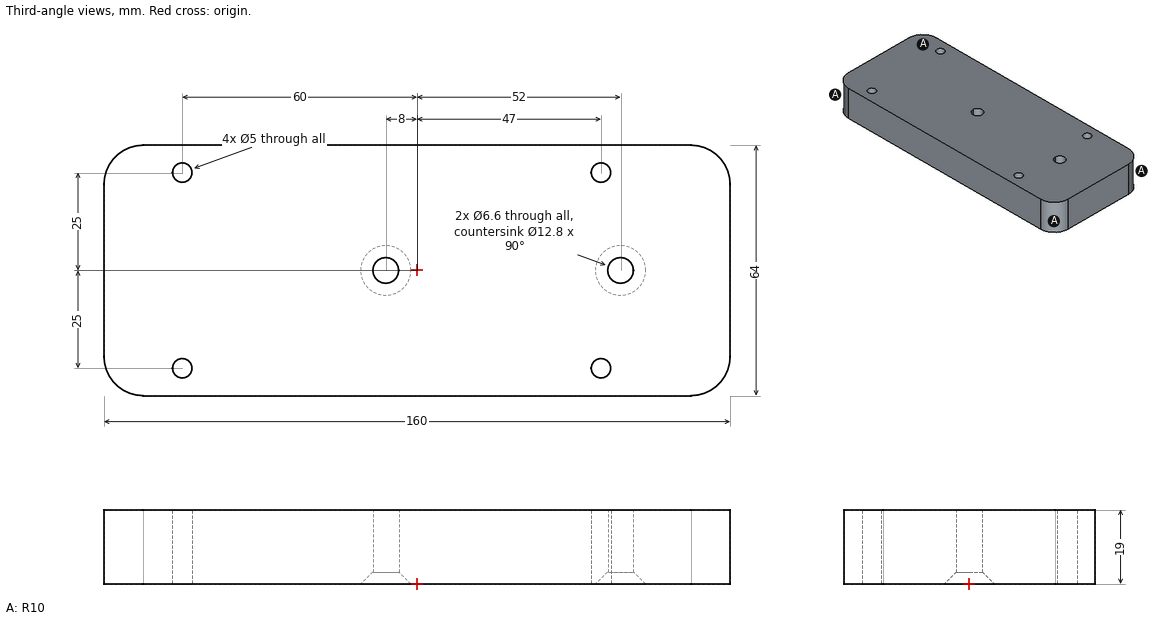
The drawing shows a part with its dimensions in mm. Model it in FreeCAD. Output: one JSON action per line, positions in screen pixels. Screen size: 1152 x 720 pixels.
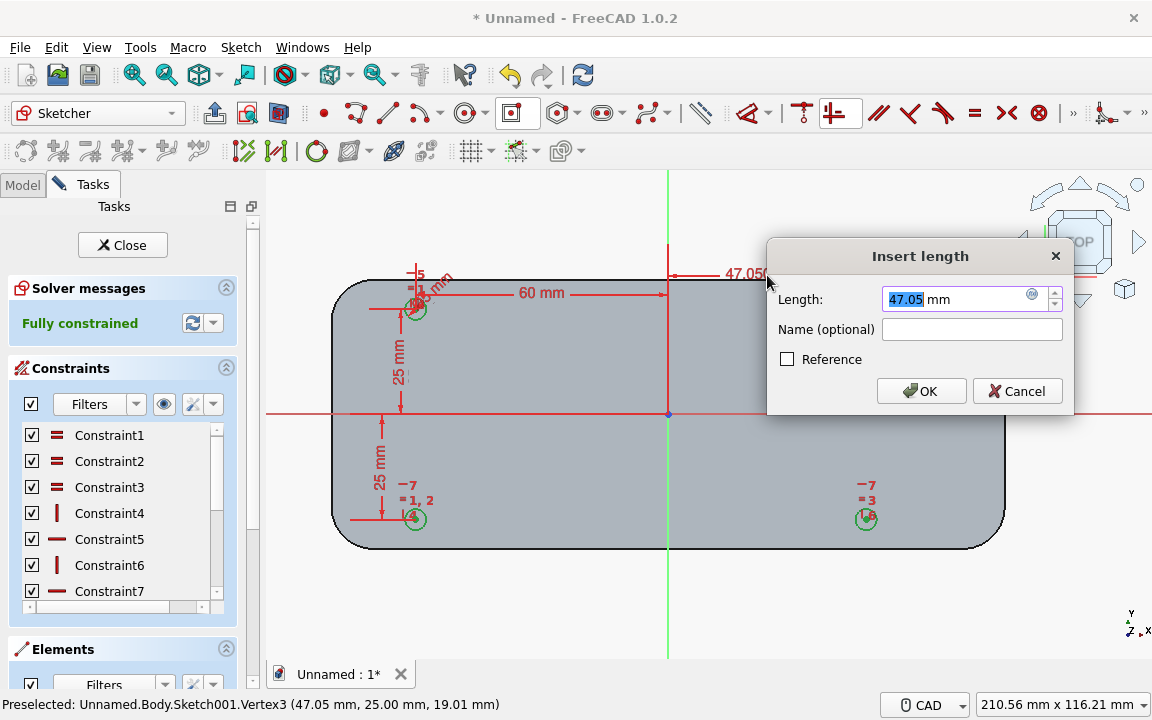
{"action": "type", "text": "47"}
{"action": "key", "text": "Return"}
{"action": "key", "text": "Escape"}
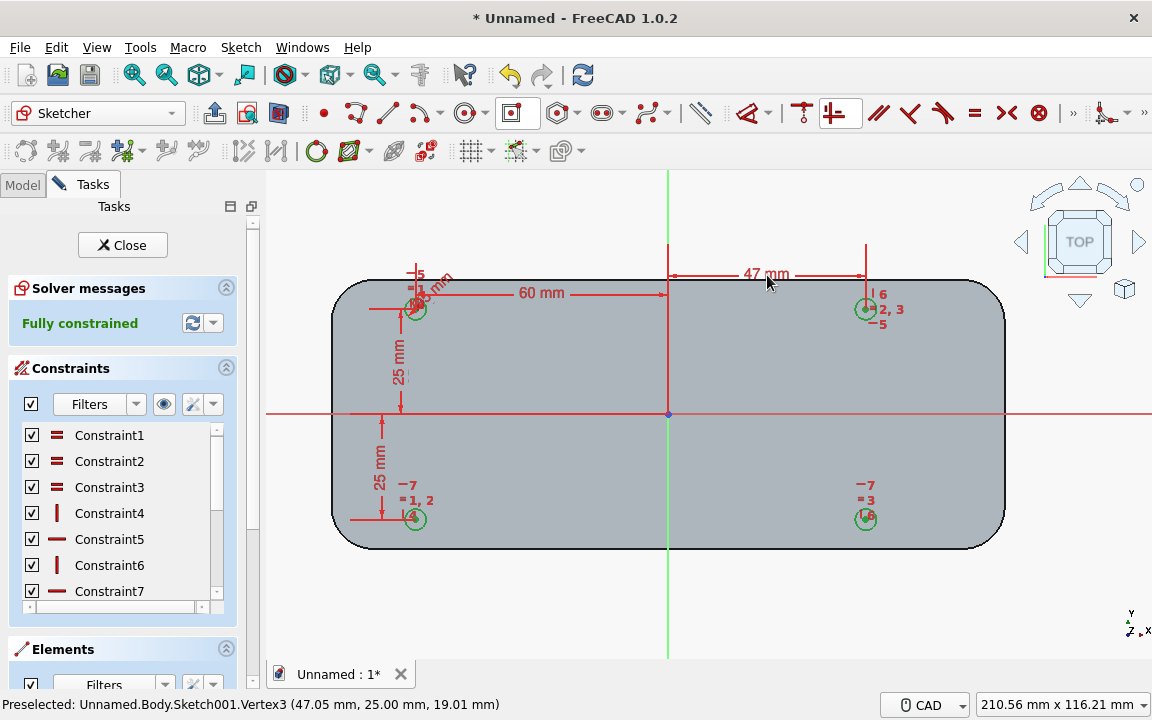
{"action": "left_click", "coordinate": [123, 245]}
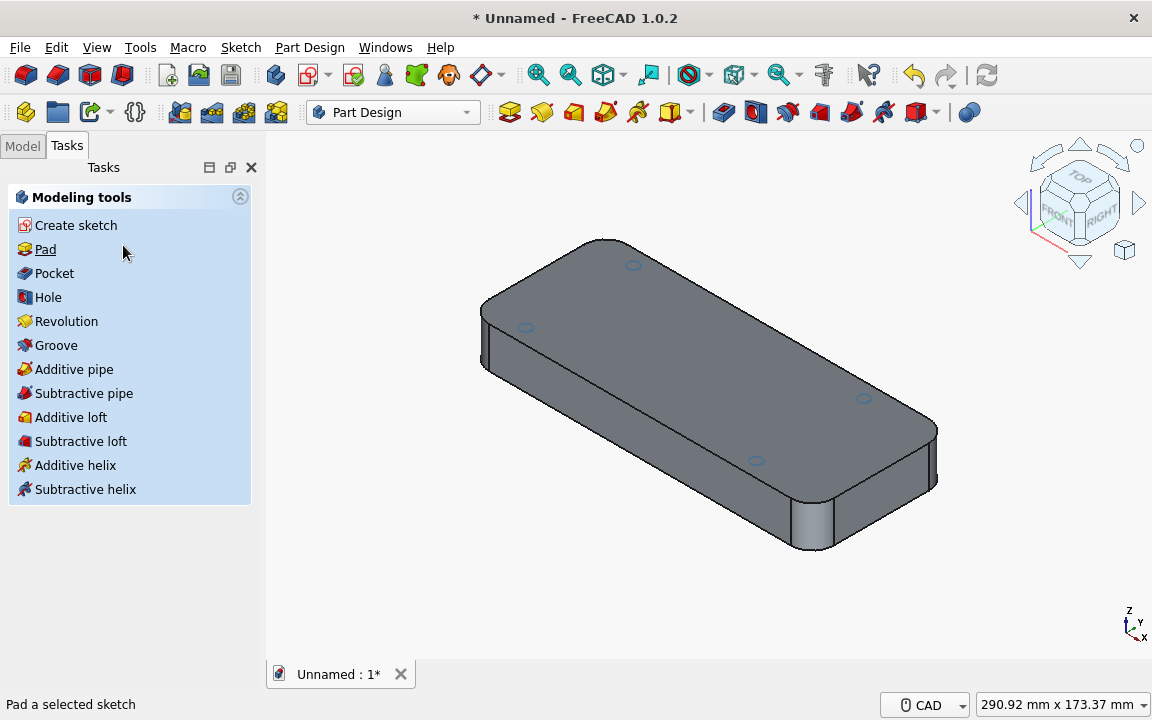
{"action": "left_click", "coordinate": [756, 112]}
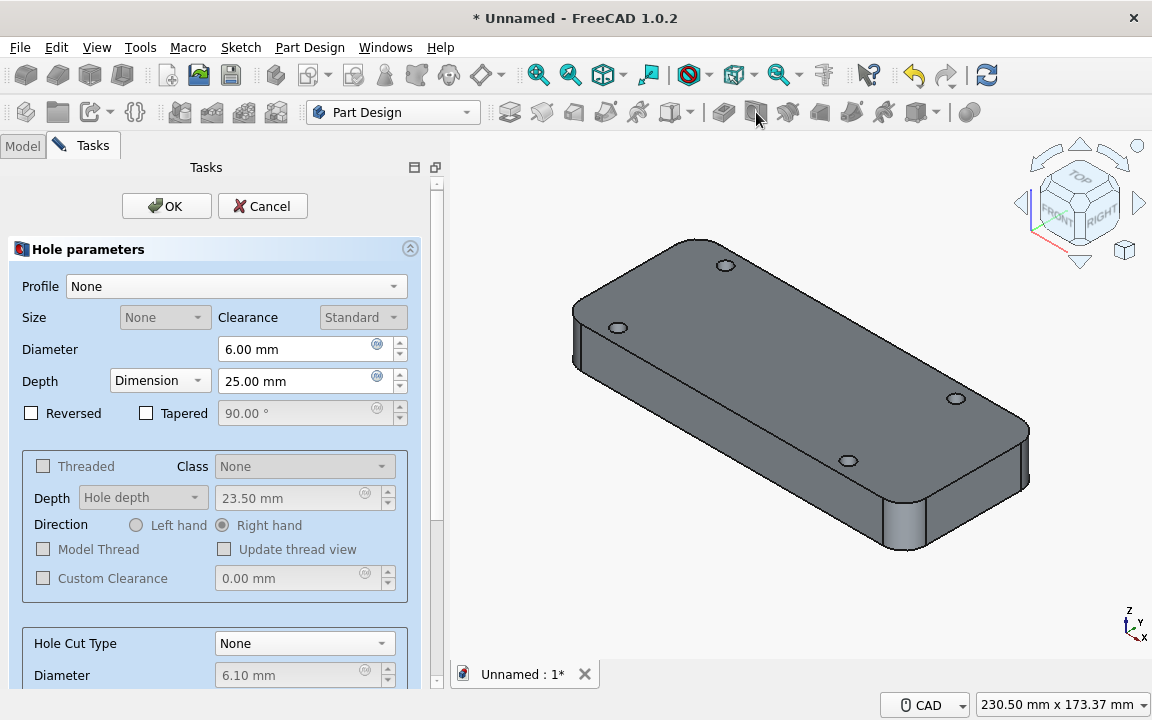
{"action": "triple_click", "coordinate": [305, 349]}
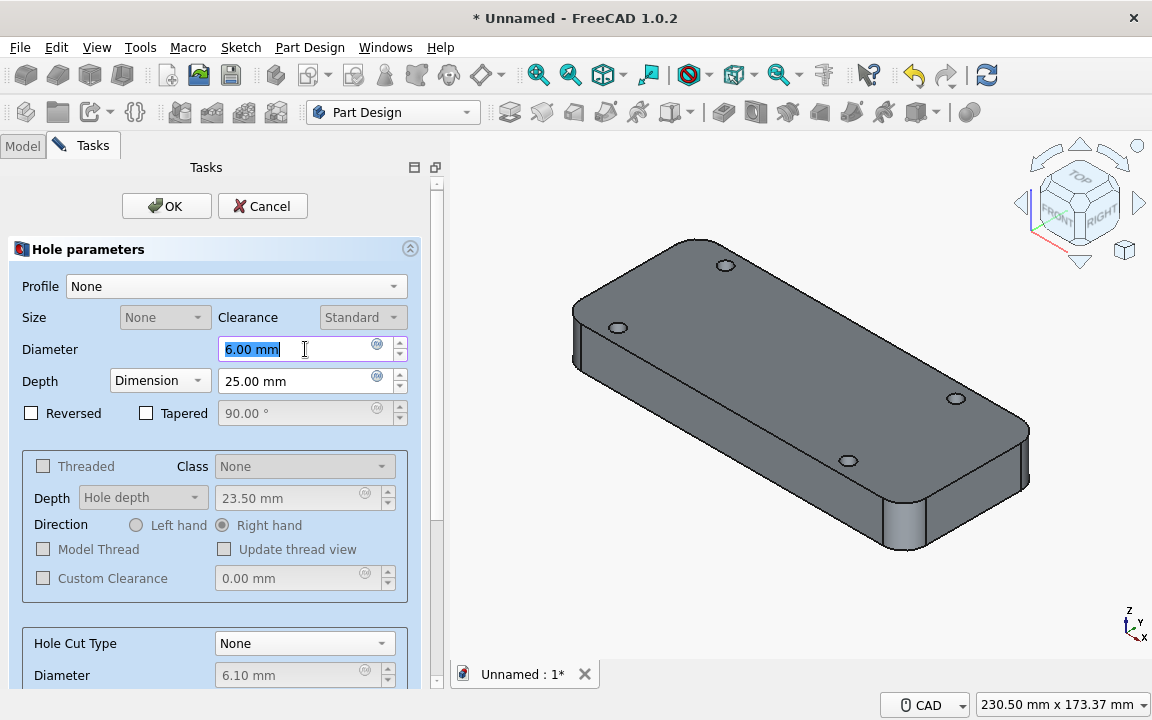
{"action": "type", "text": "5"}
{"action": "key", "text": "Tab"}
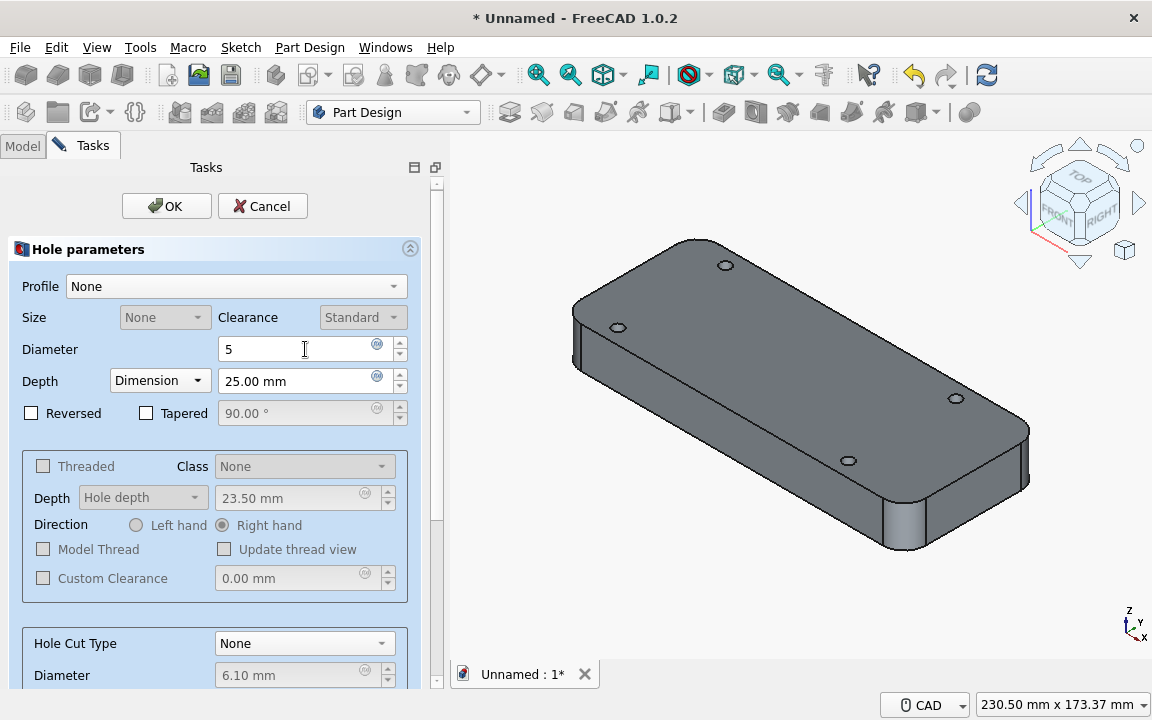
{"action": "left_click", "coordinate": [161, 380]}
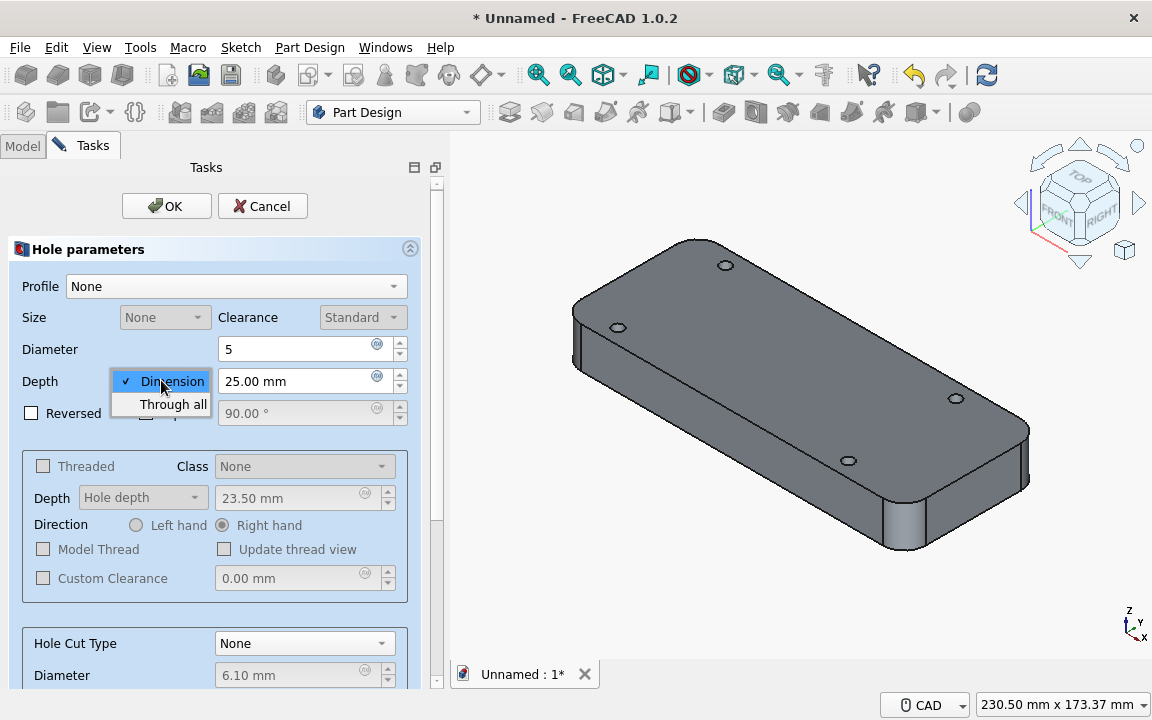
{"action": "left_click", "coordinate": [160, 404]}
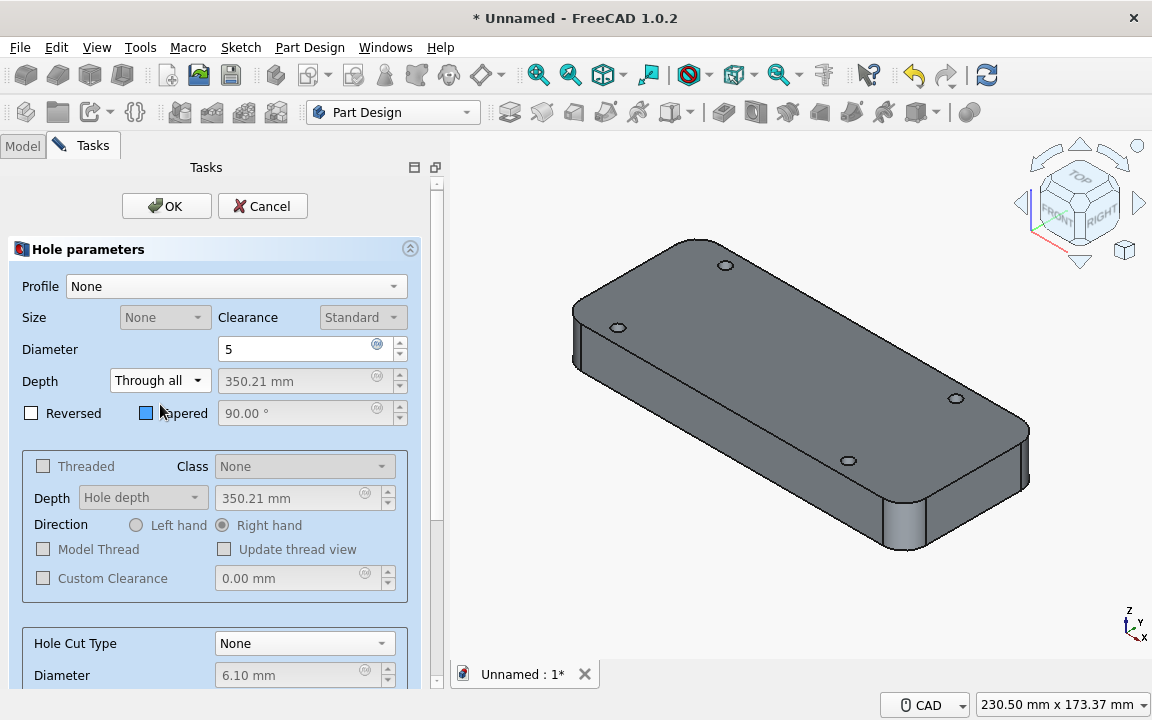
{"action": "left_click", "coordinate": [167, 206]}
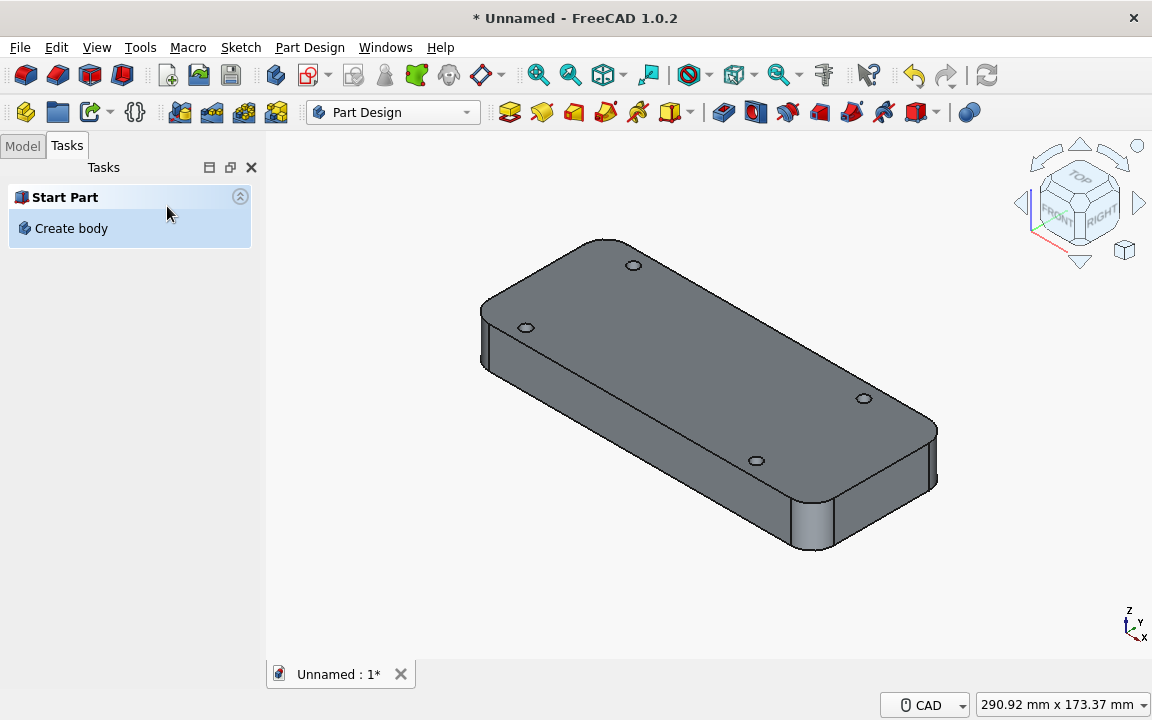
{"action": "key", "text": "5"}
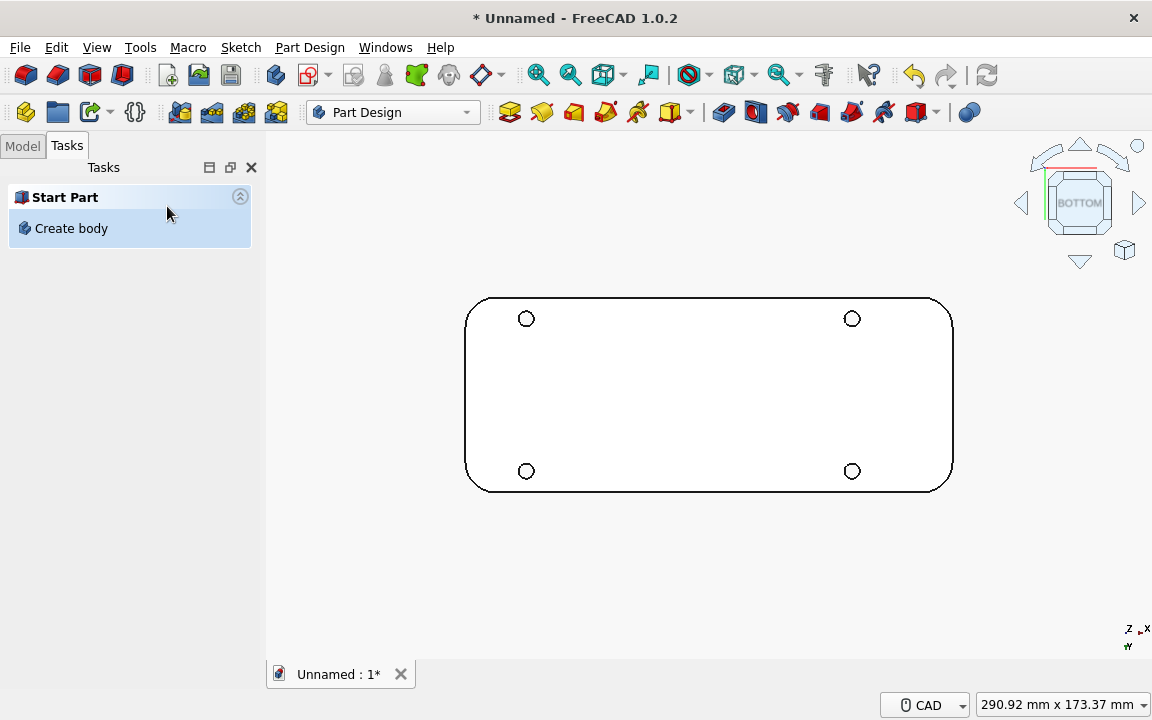
{"action": "left_click", "coordinate": [779, 394]}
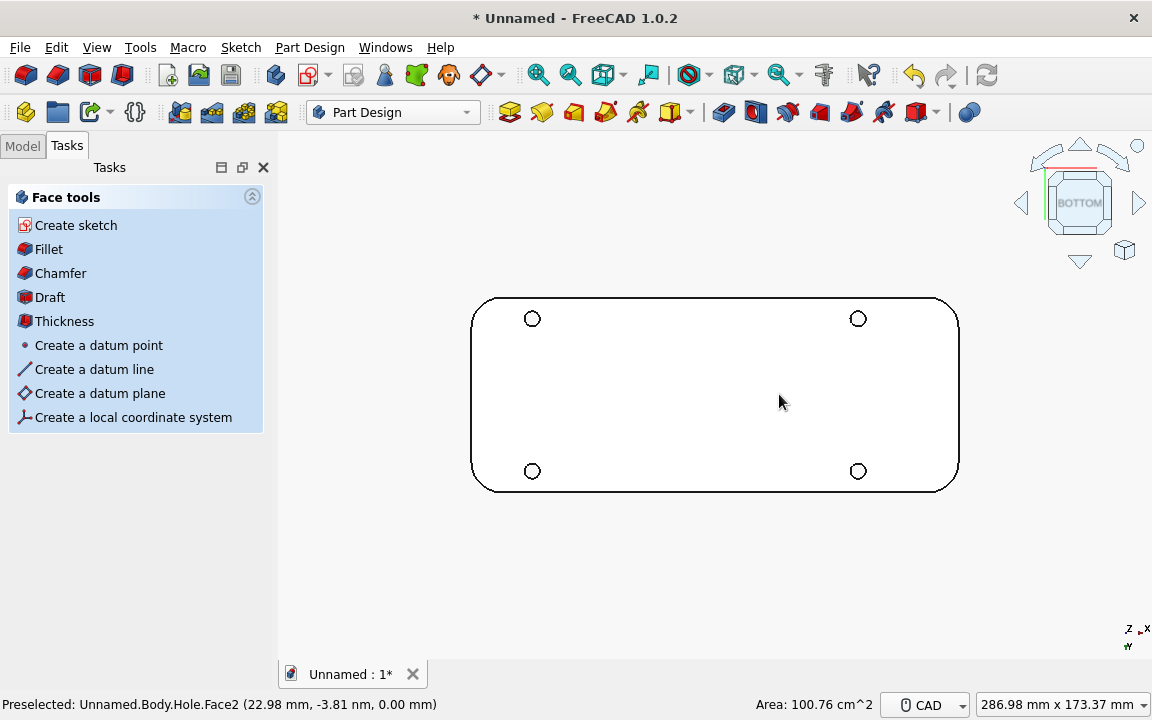
{"action": "left_click", "coordinate": [308, 76]}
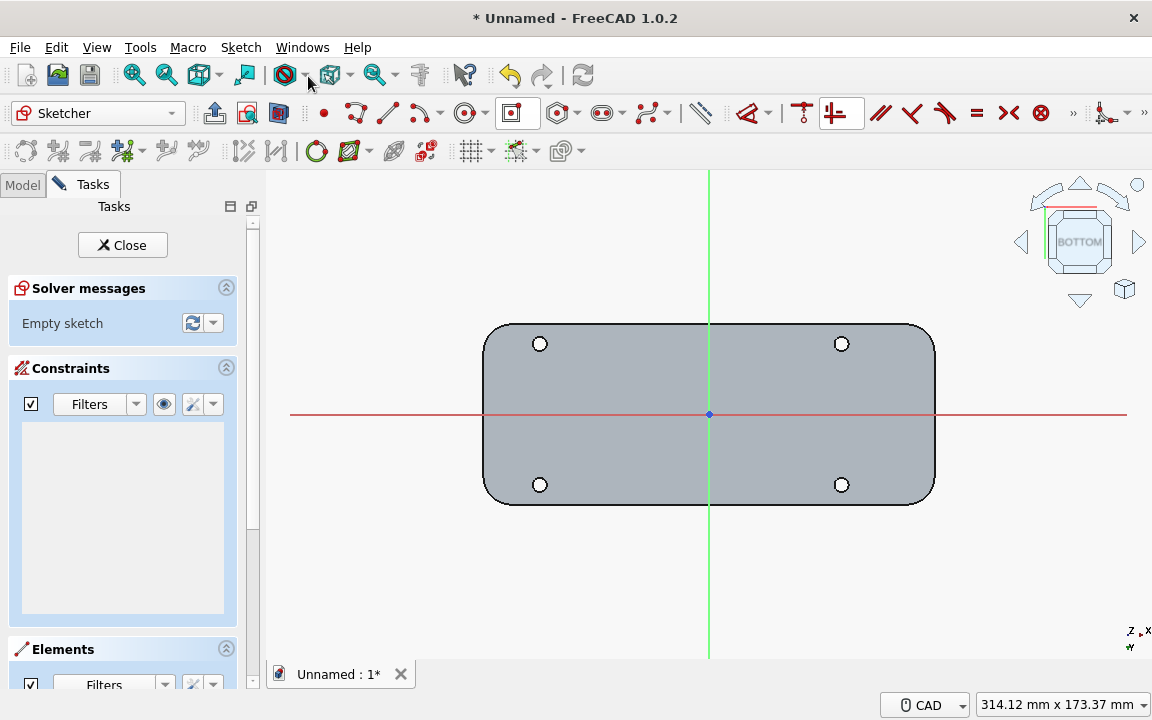
{"action": "scroll", "coordinate": [847, 415], "scroll_direction": "up", "scroll_amount": 5}